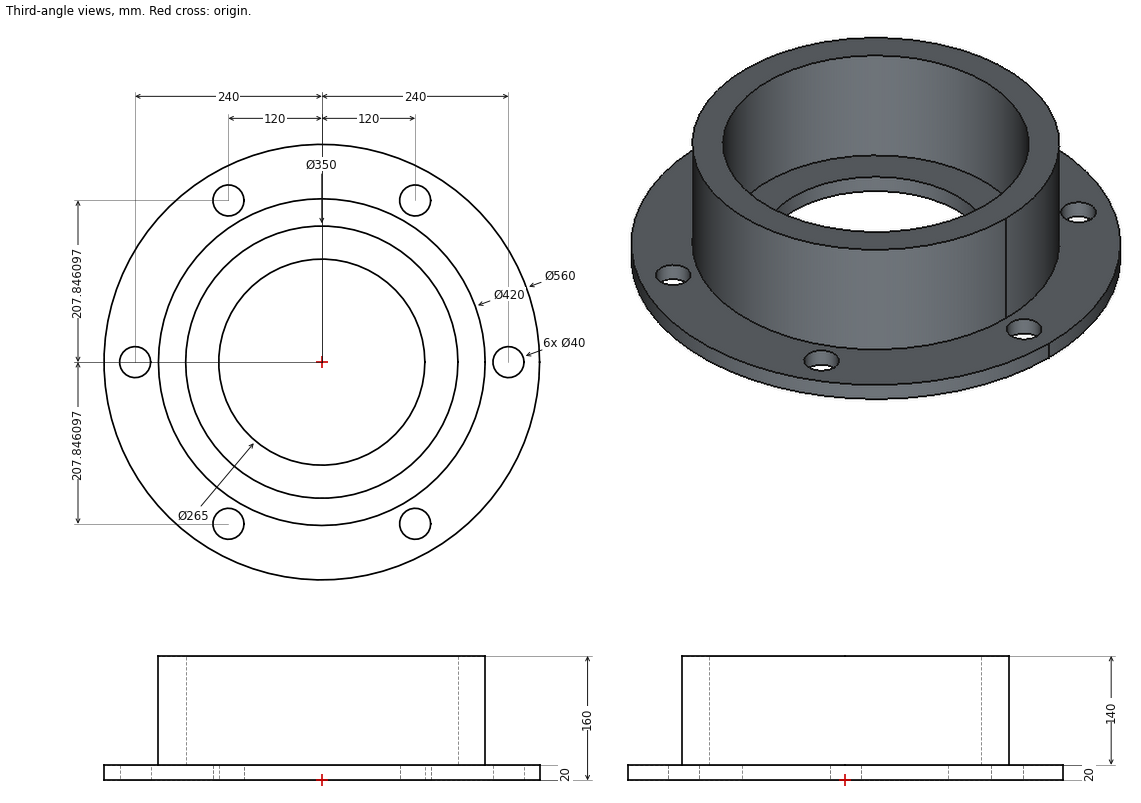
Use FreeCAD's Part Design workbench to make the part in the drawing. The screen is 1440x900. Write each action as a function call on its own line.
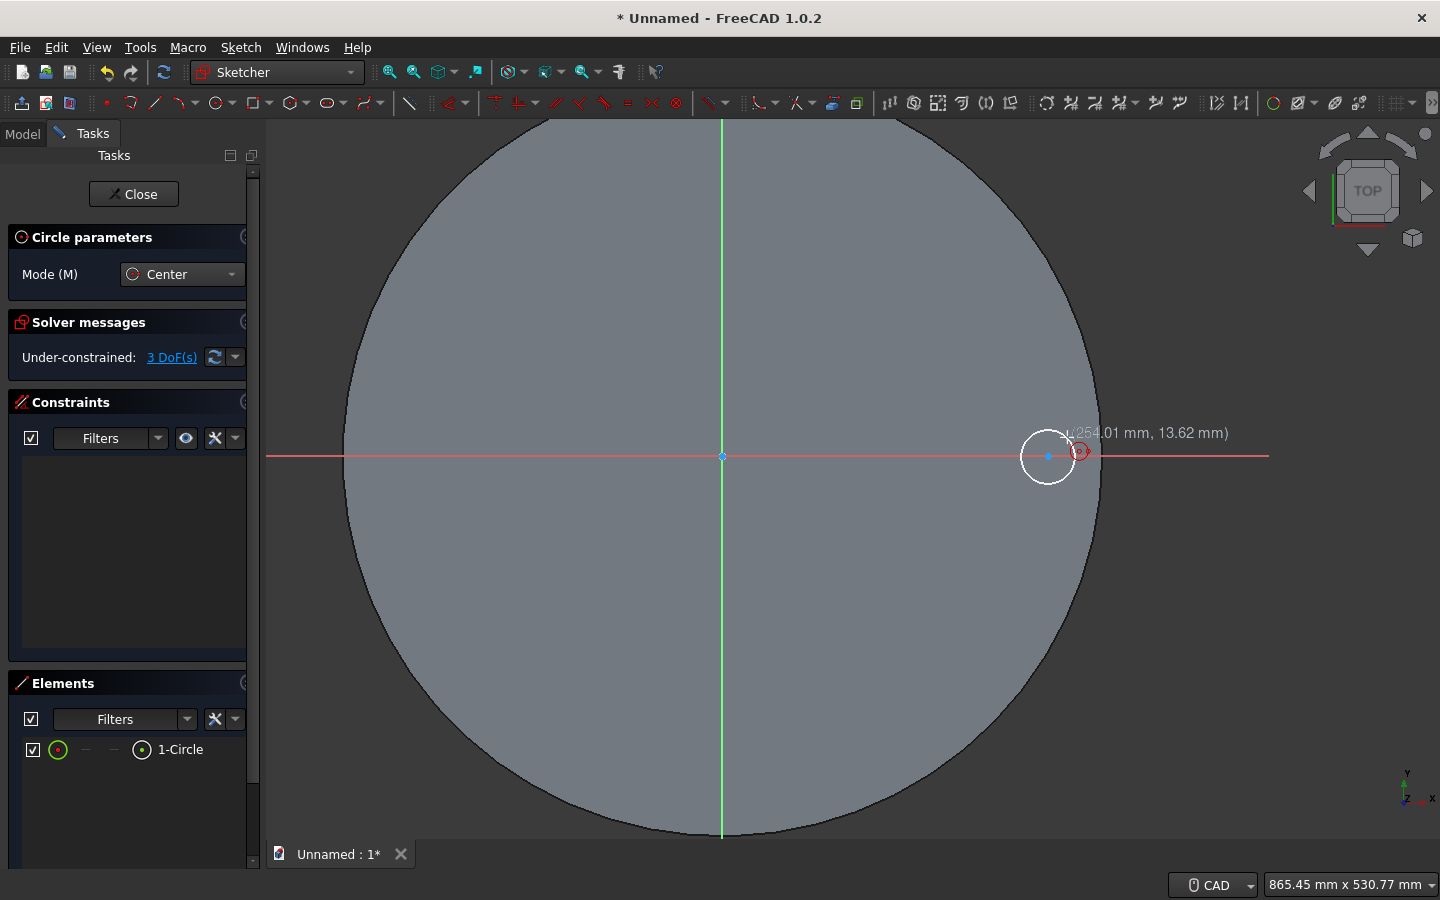
click(397, 456)
click(416, 437)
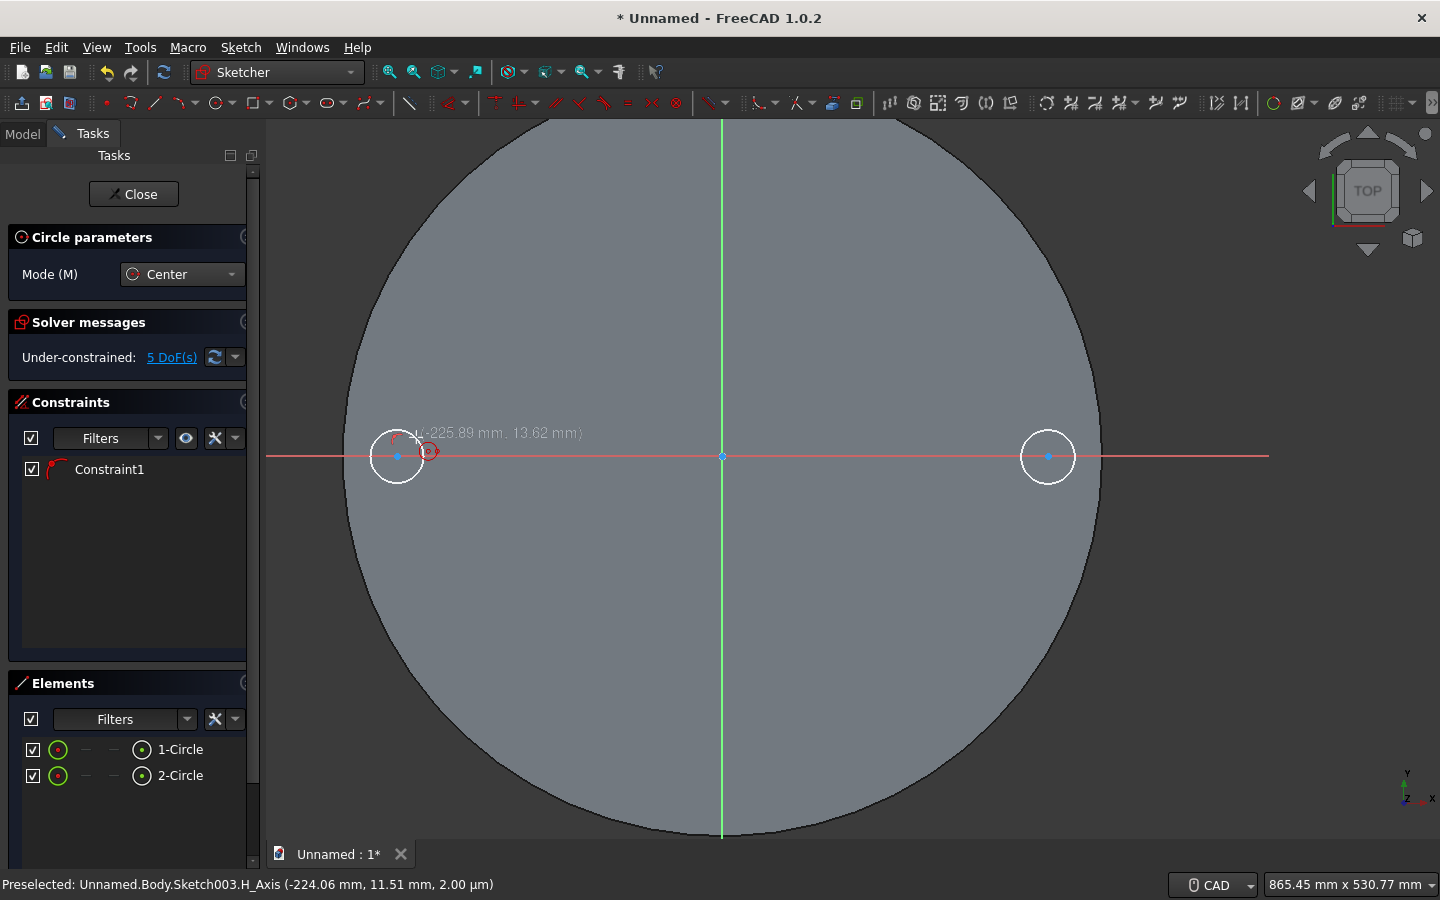
click(560, 175)
click(579, 155)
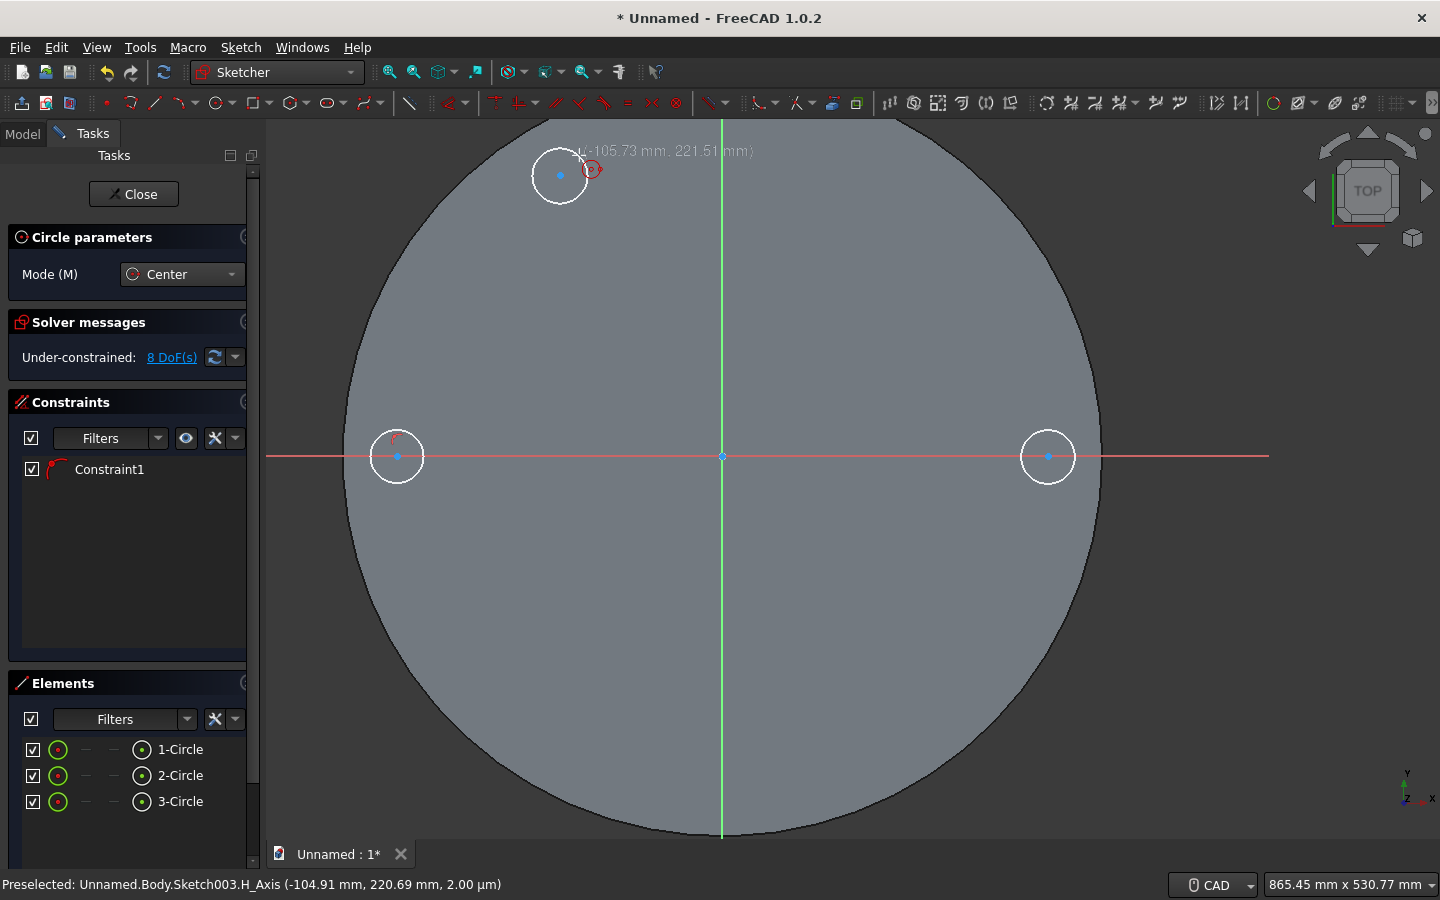
click(885, 175)
click(904, 155)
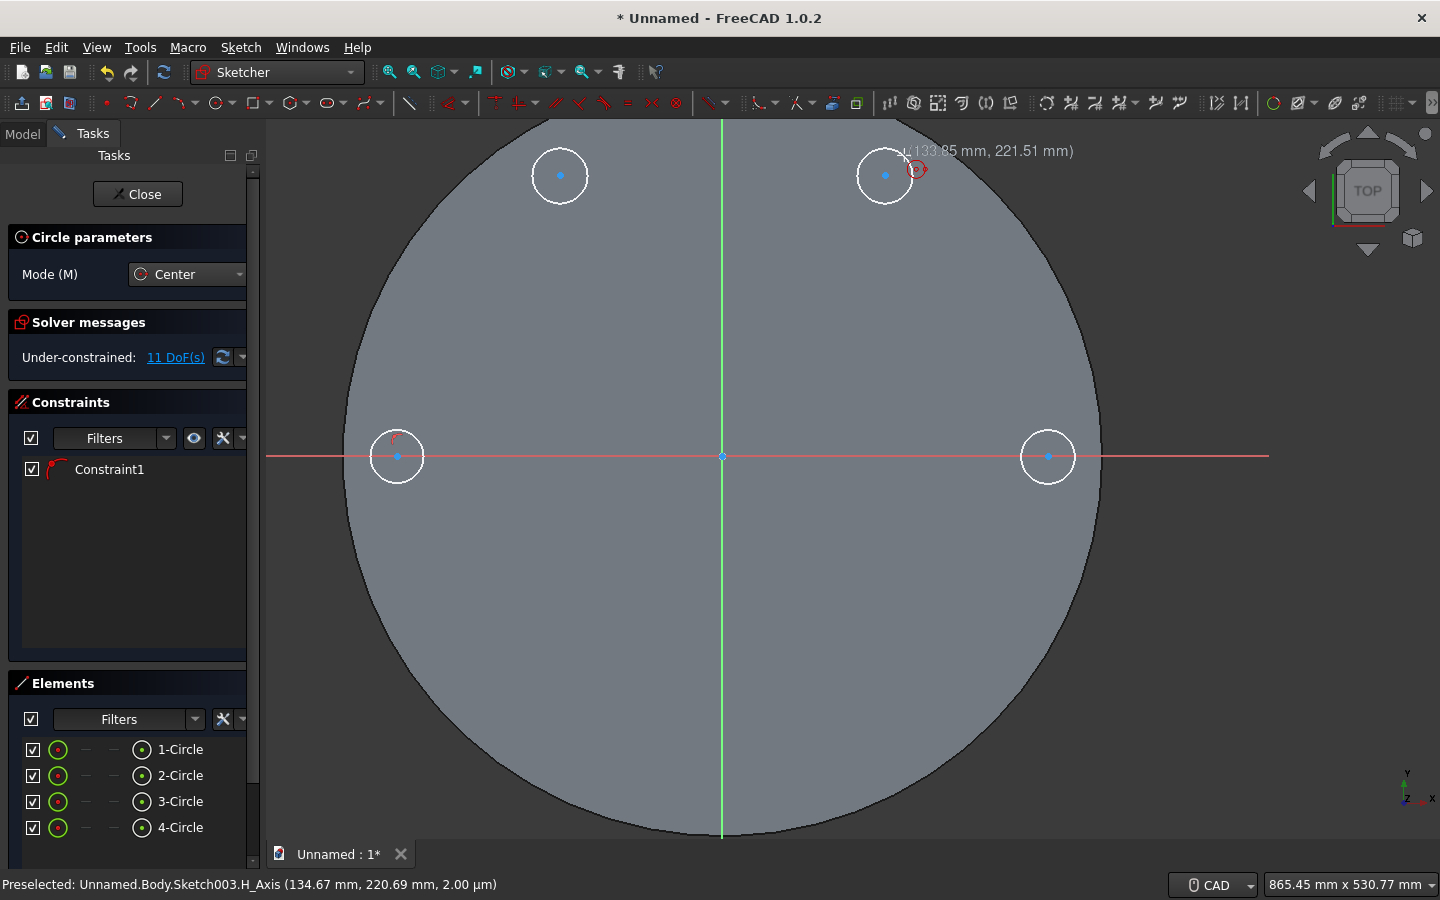
click(560, 738)
click(579, 719)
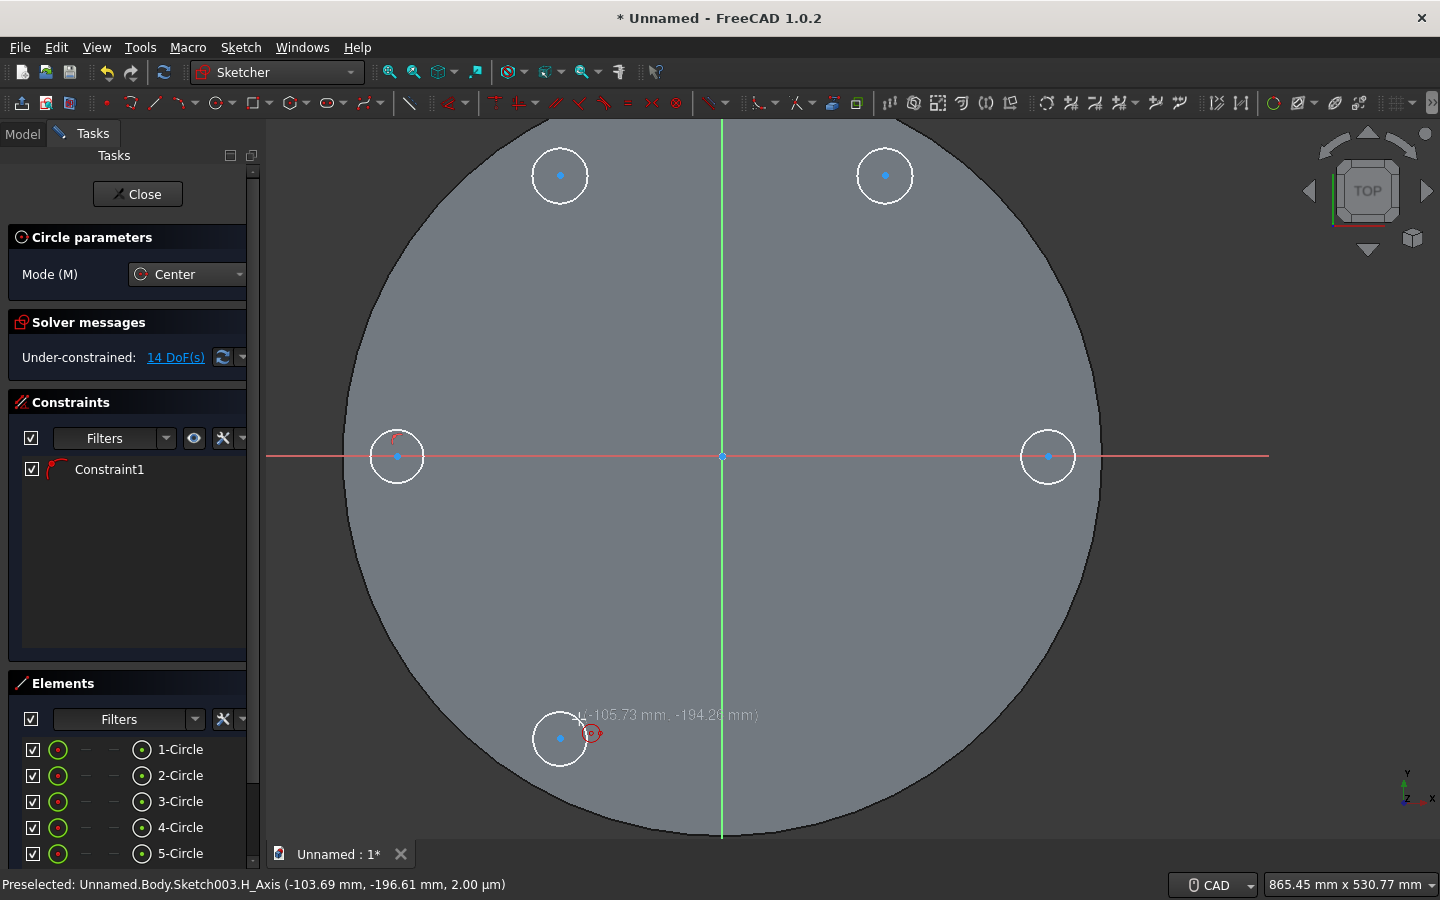
click(885, 738)
click(904, 719)
key(Escape)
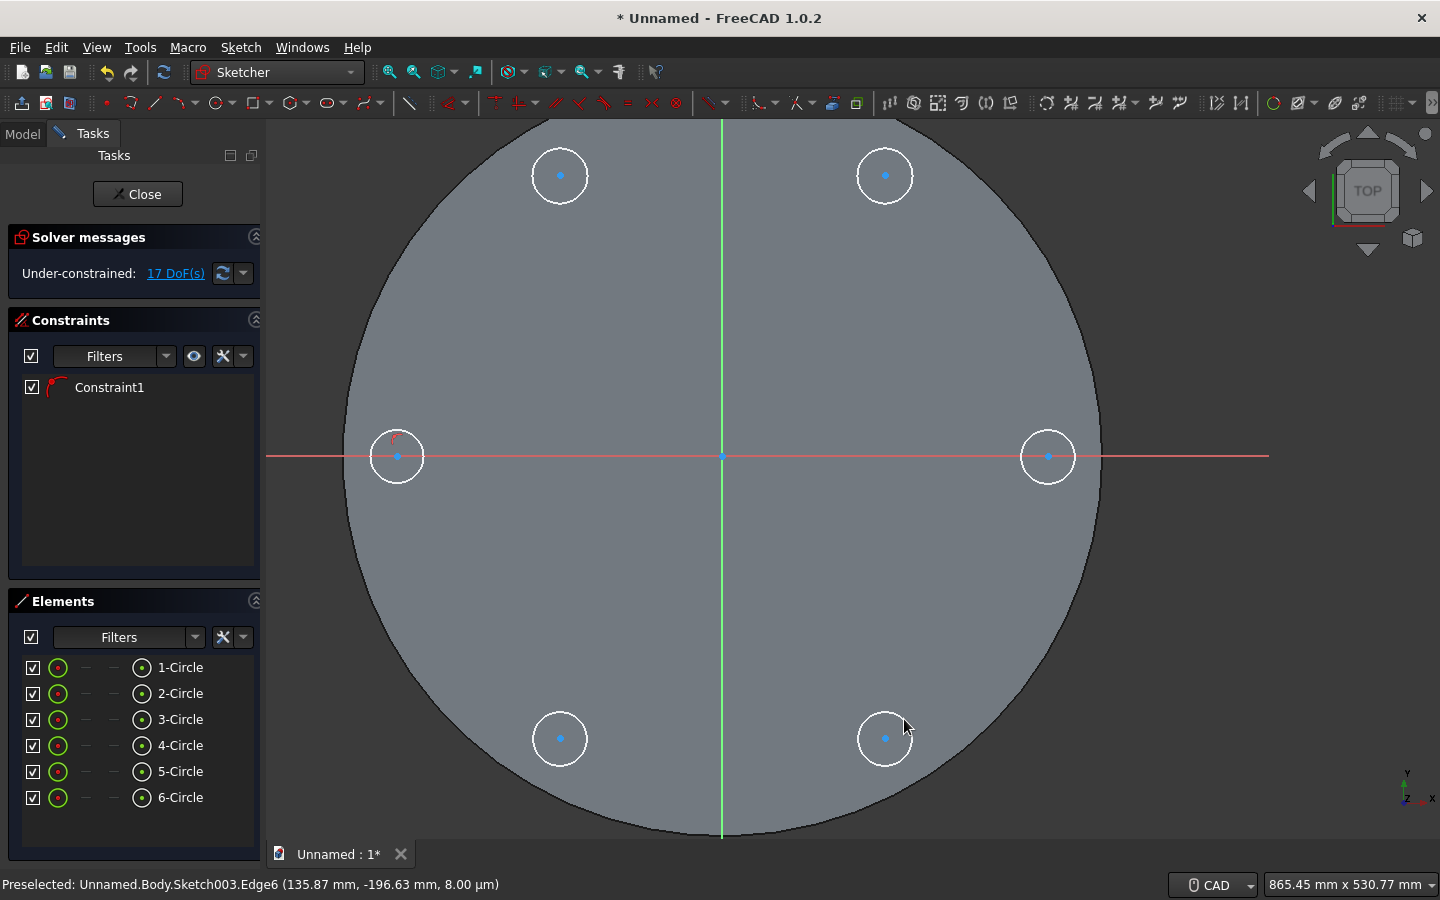
click(1067, 438)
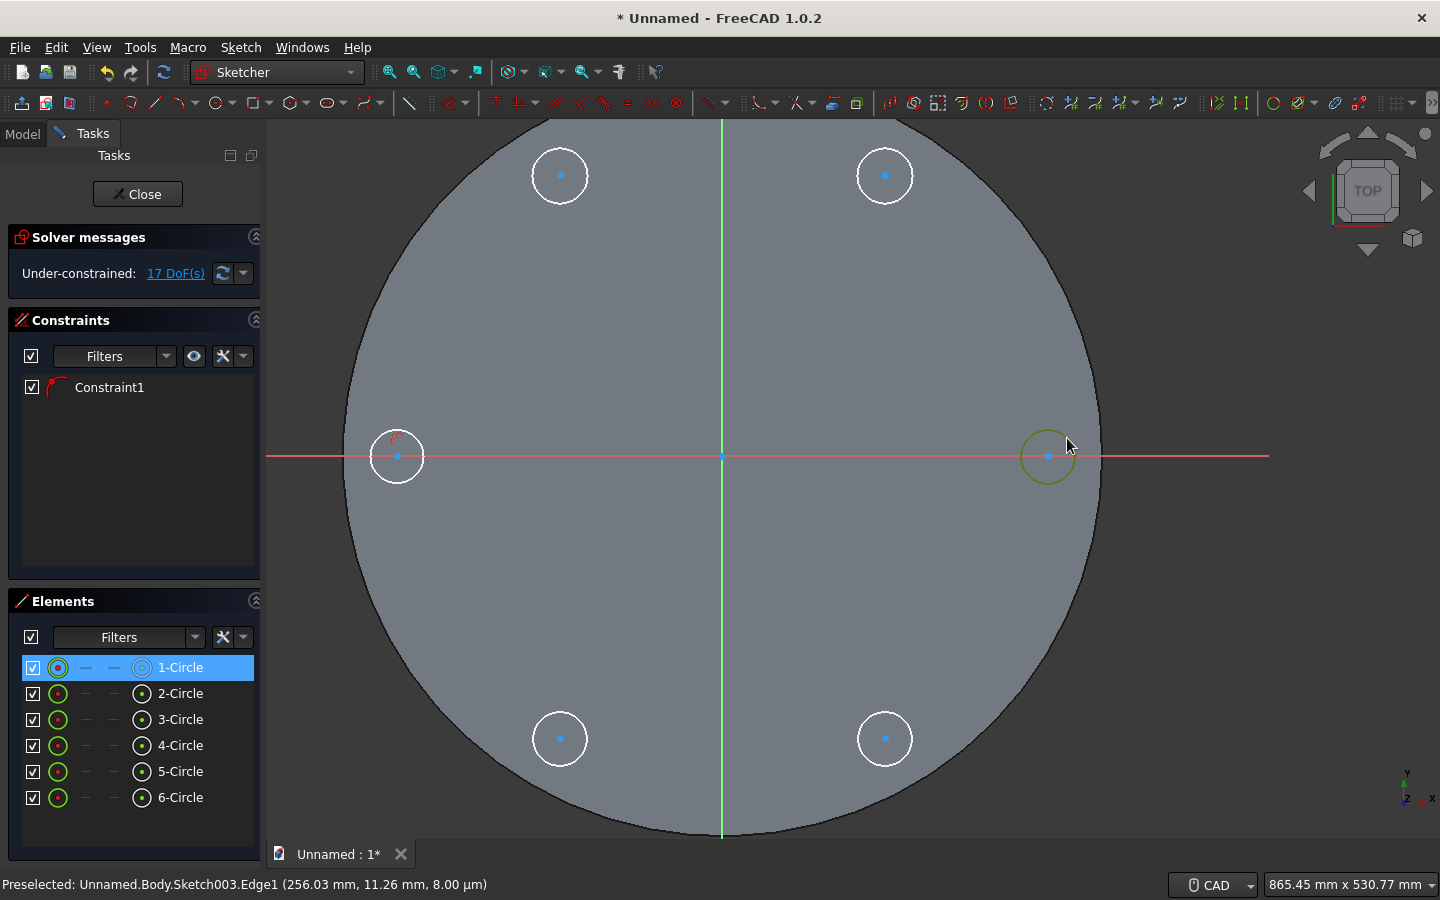
click(416, 438)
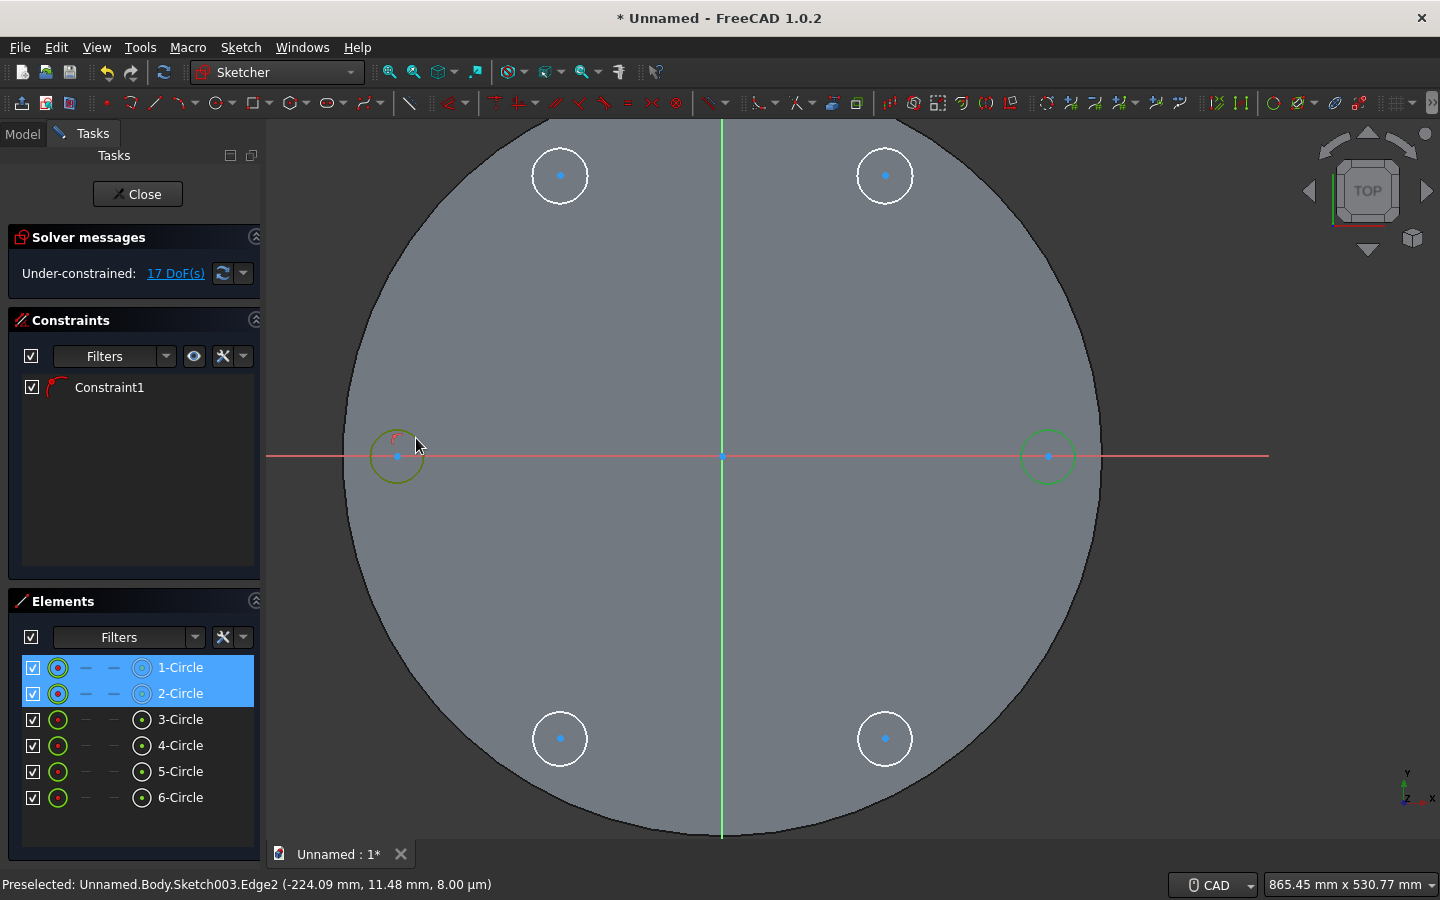
click(579, 156)